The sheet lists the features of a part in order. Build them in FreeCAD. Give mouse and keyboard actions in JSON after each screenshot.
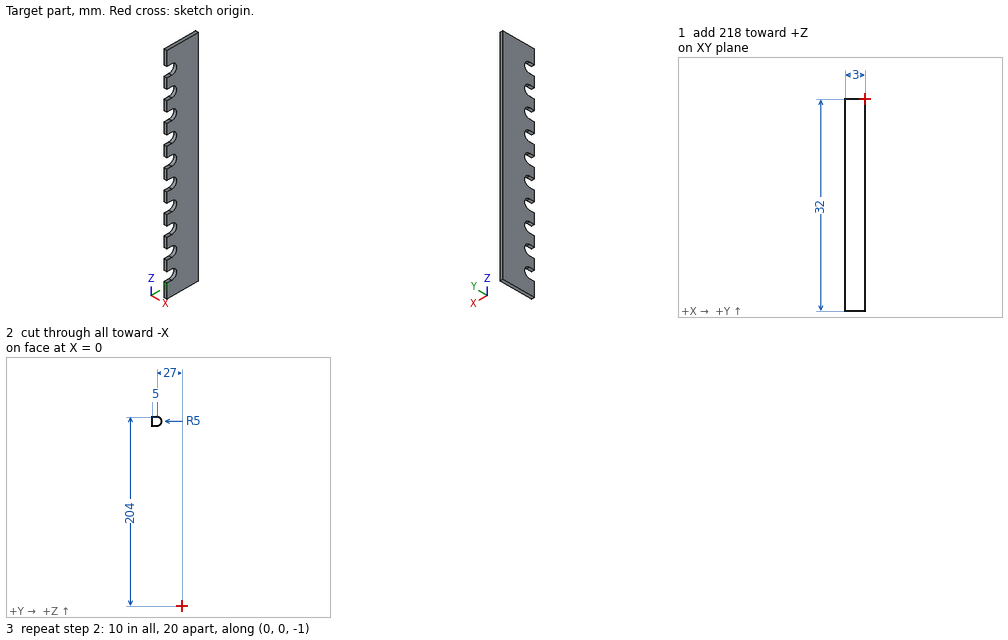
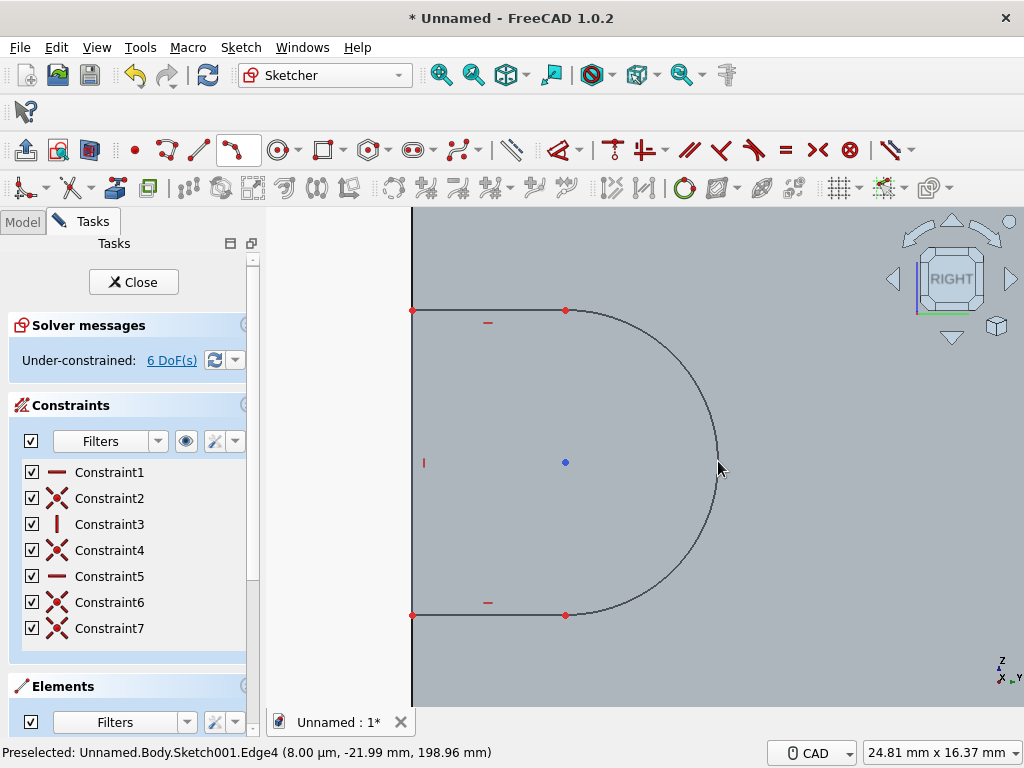
{"action": "left_click", "coordinate": [519, 310]}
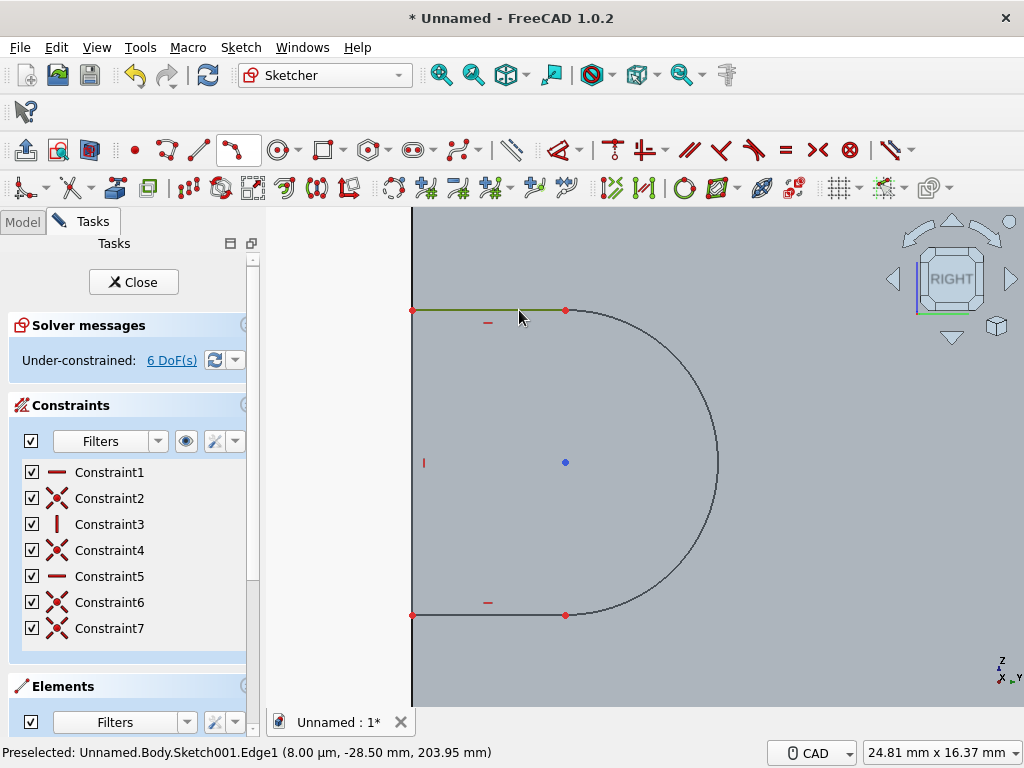
{"action": "left_click", "coordinate": [689, 552]}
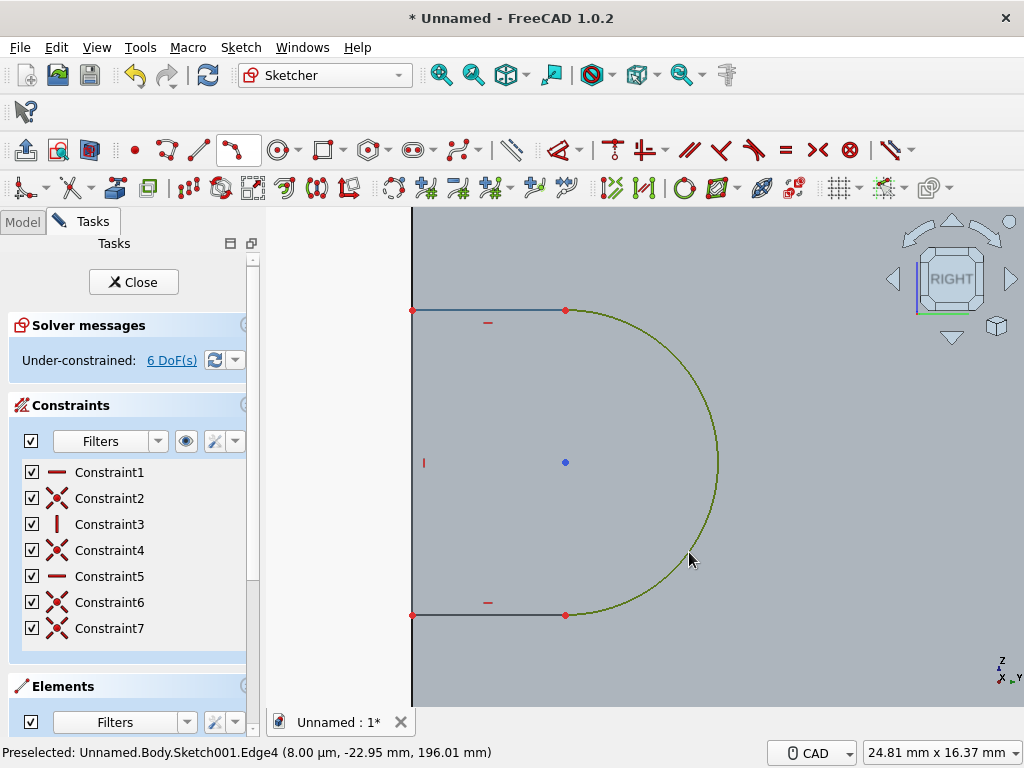
{"action": "left_click", "coordinate": [754, 150]}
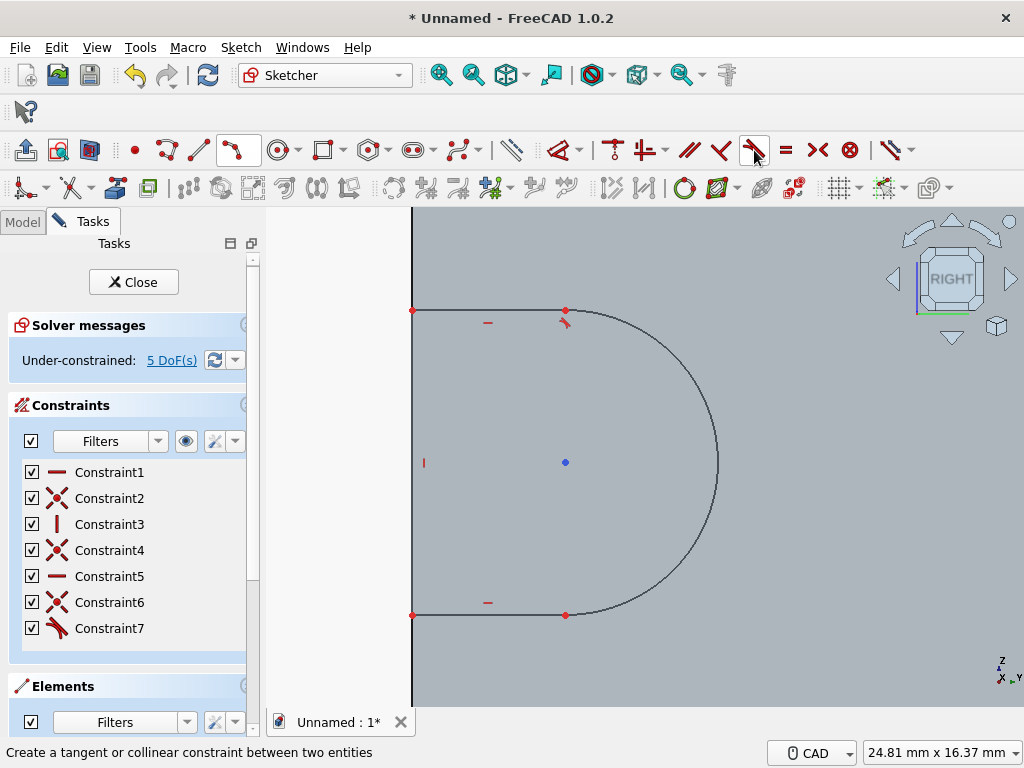
{"action": "left_click", "coordinate": [458, 615]}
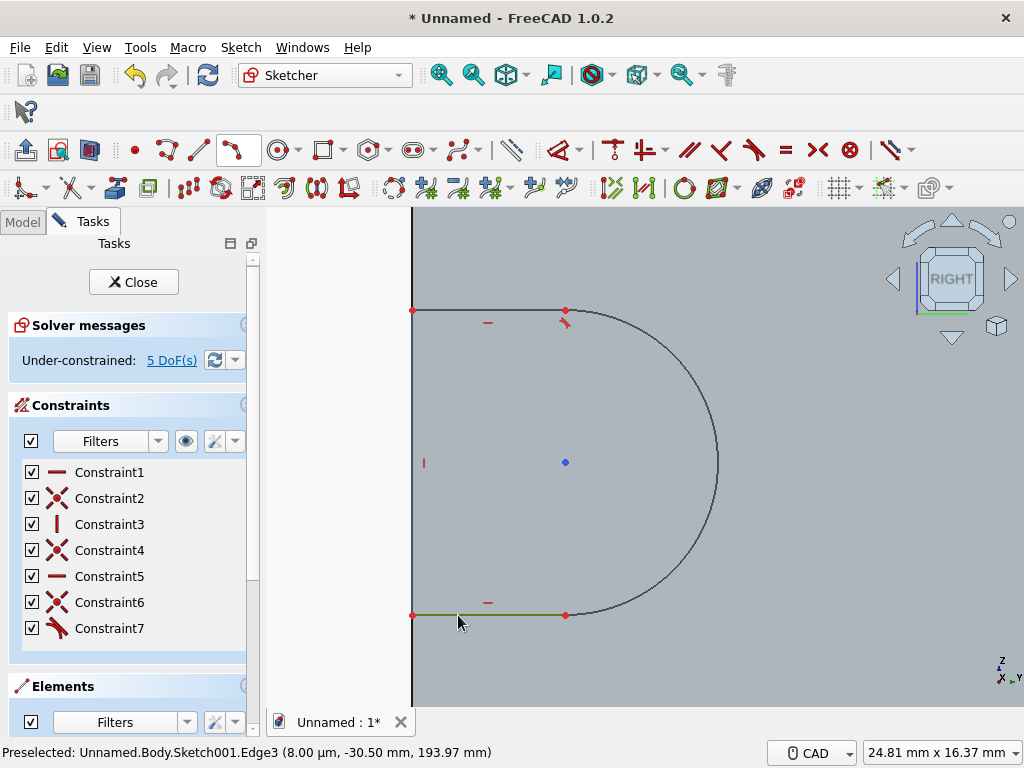
{"action": "left_click", "coordinate": [689, 552]}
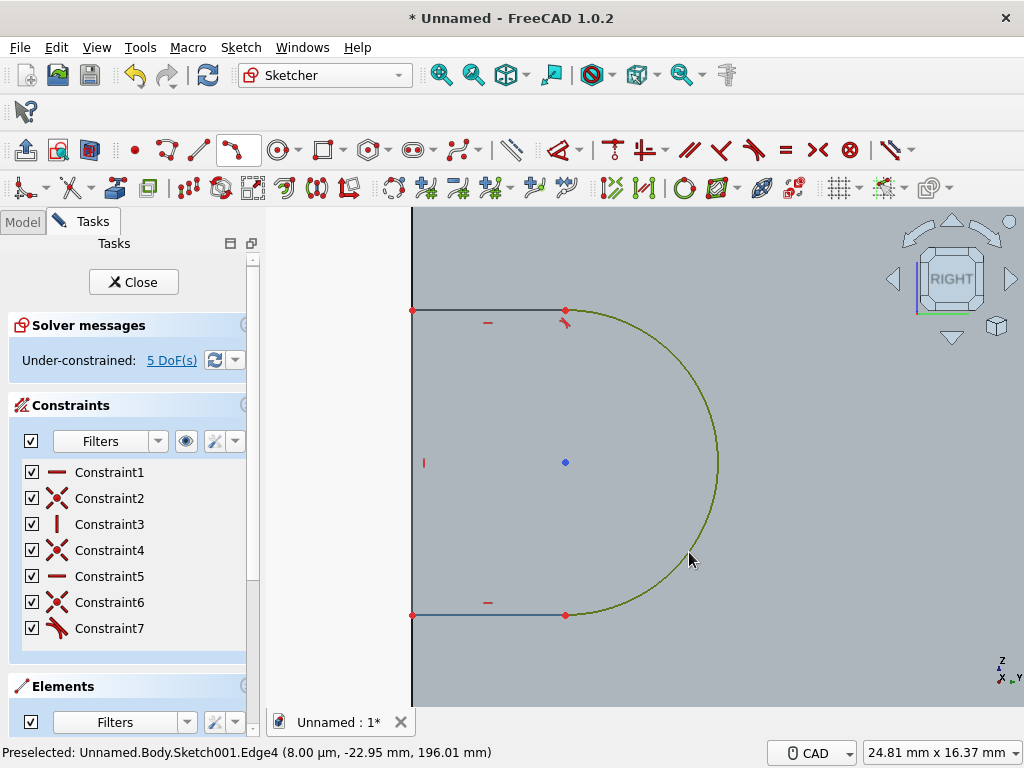
{"action": "left_click", "coordinate": [754, 150]}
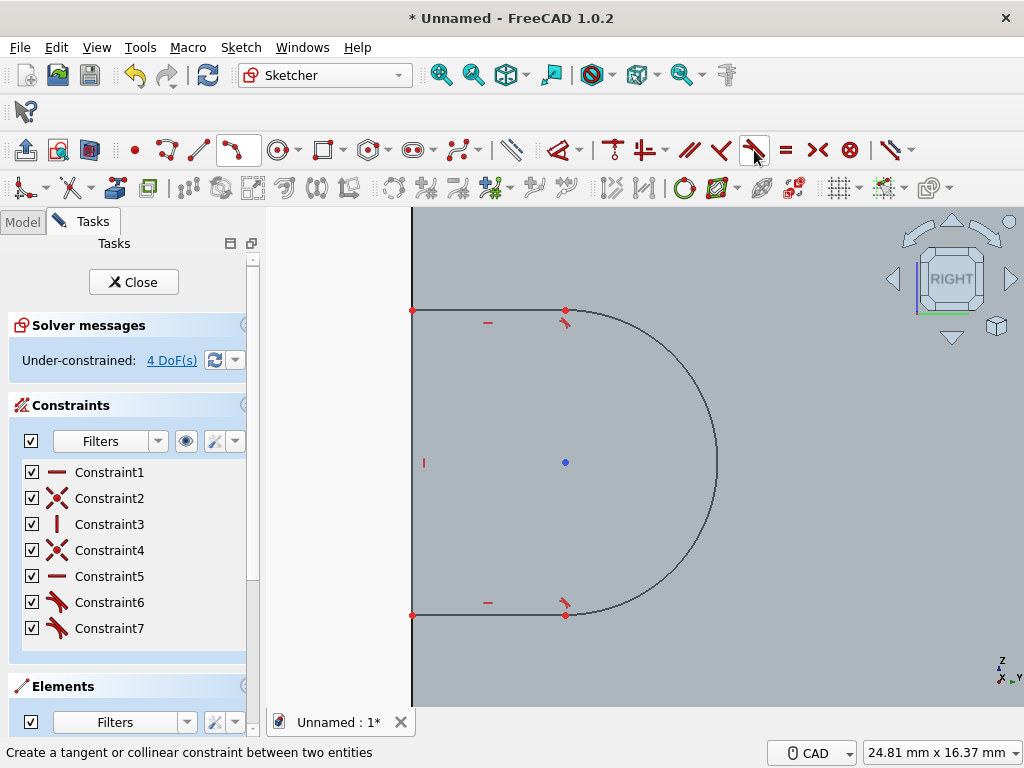
{"action": "left_click", "coordinate": [558, 150]}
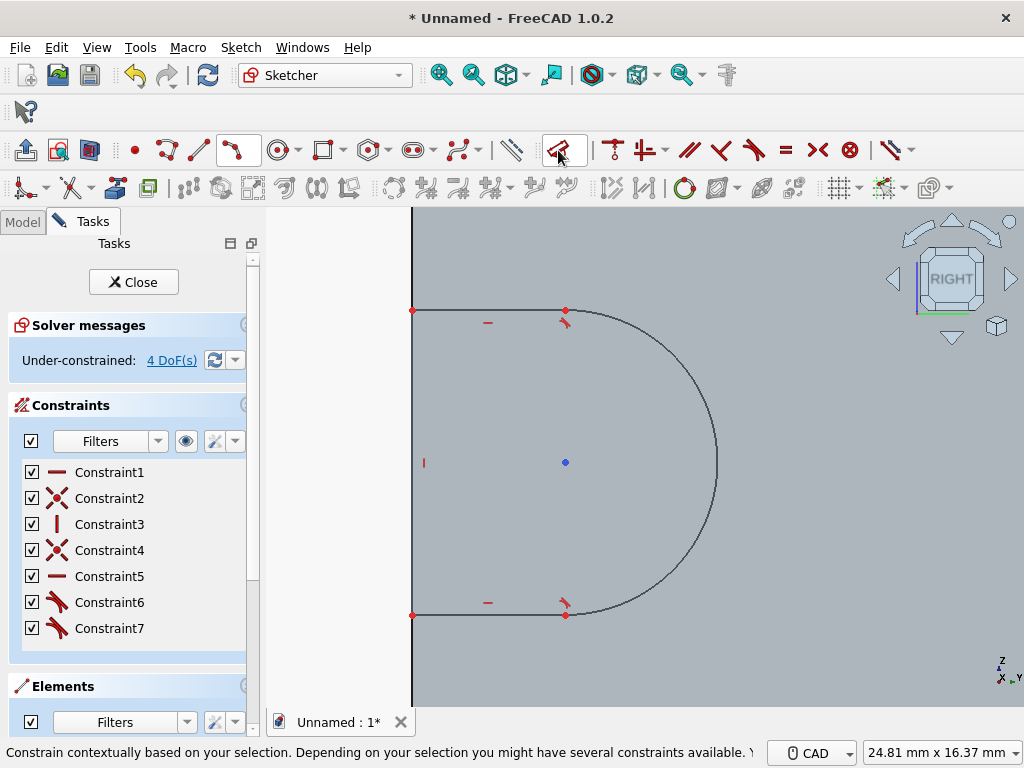
{"action": "left_click", "coordinate": [688, 552]}
{"action": "left_click", "coordinate": [714, 571]}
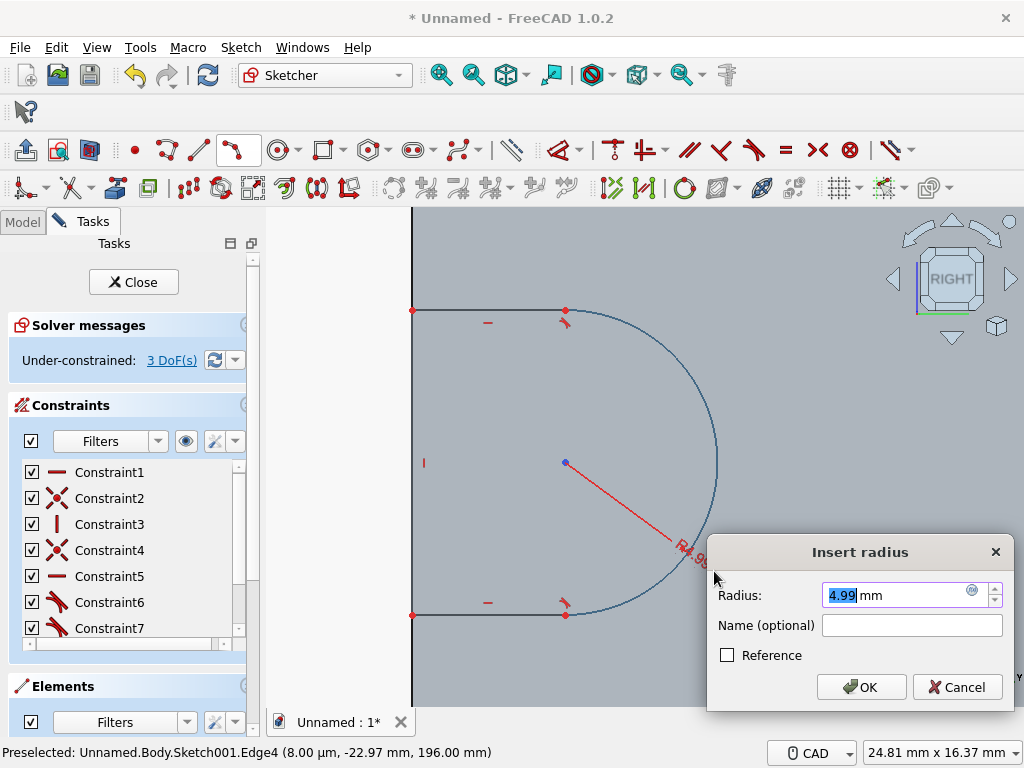
{"action": "type", "text": "5"}
{"action": "key", "text": "Return"}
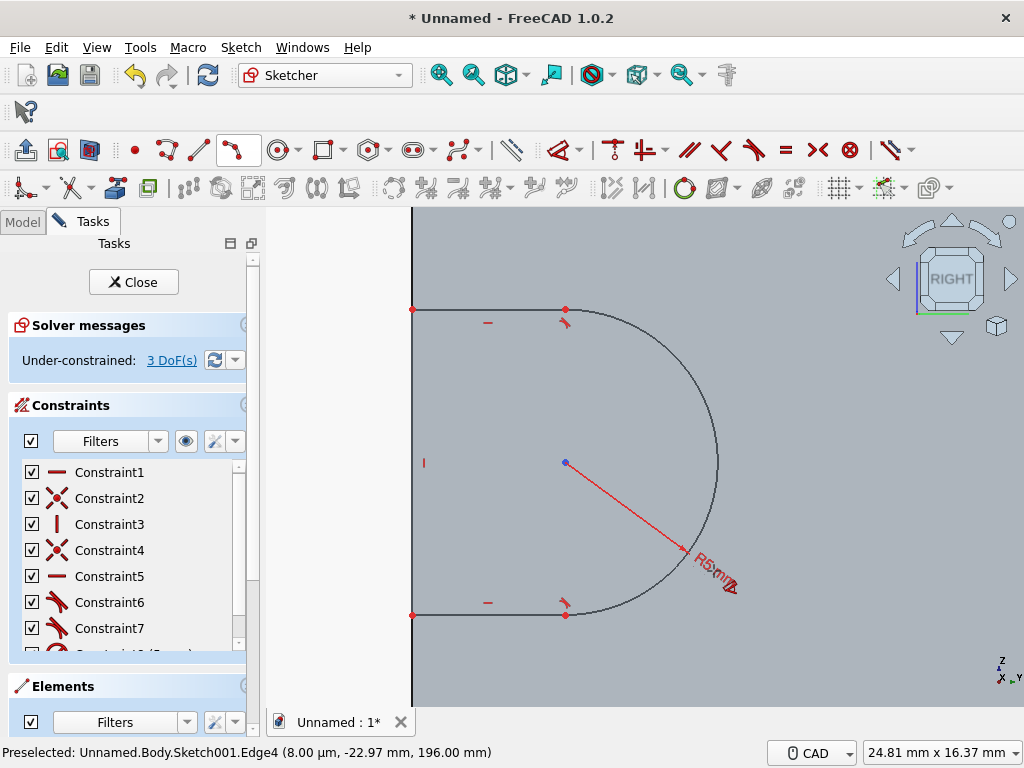
{"action": "left_click", "coordinate": [519, 310]}
{"action": "left_click", "coordinate": [489, 276]}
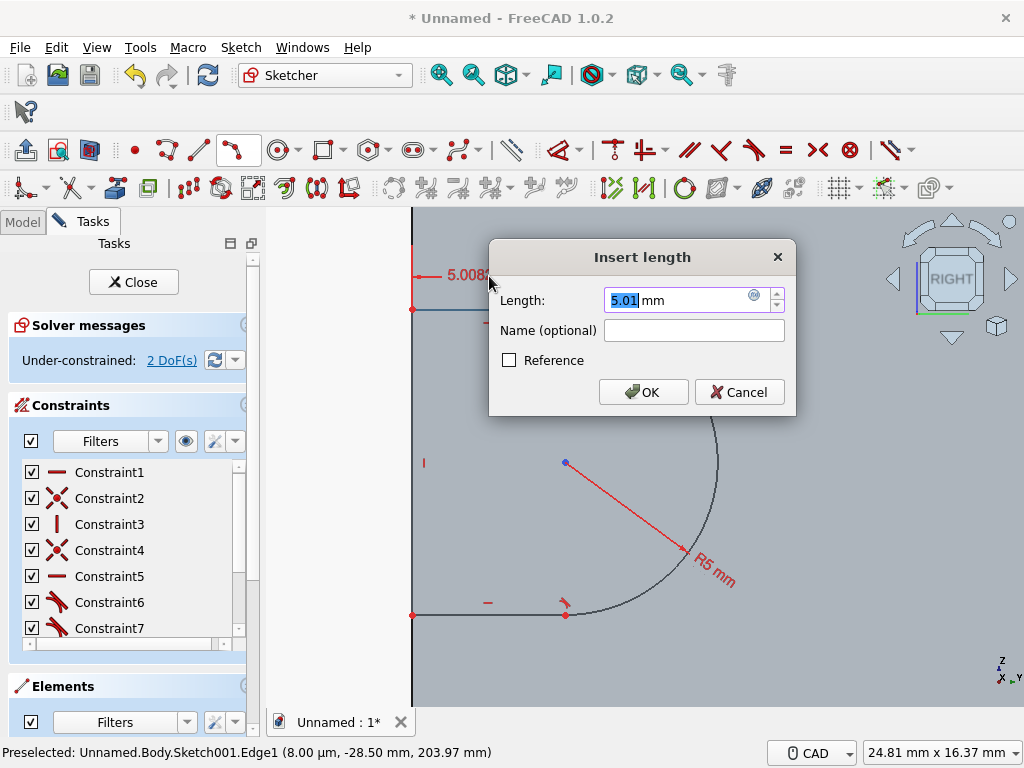
{"action": "type", "text": "5"}
{"action": "key", "text": "Return"}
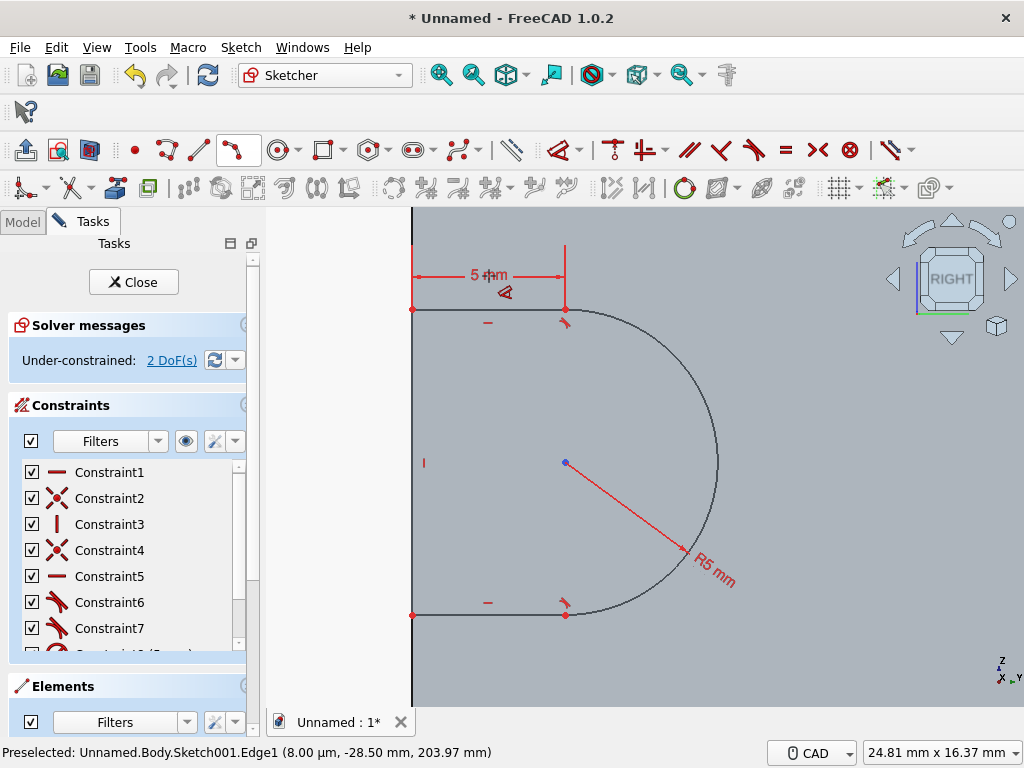
{"action": "left_click", "coordinate": [565, 310]}
{"action": "left_click", "coordinate": [712, 276]}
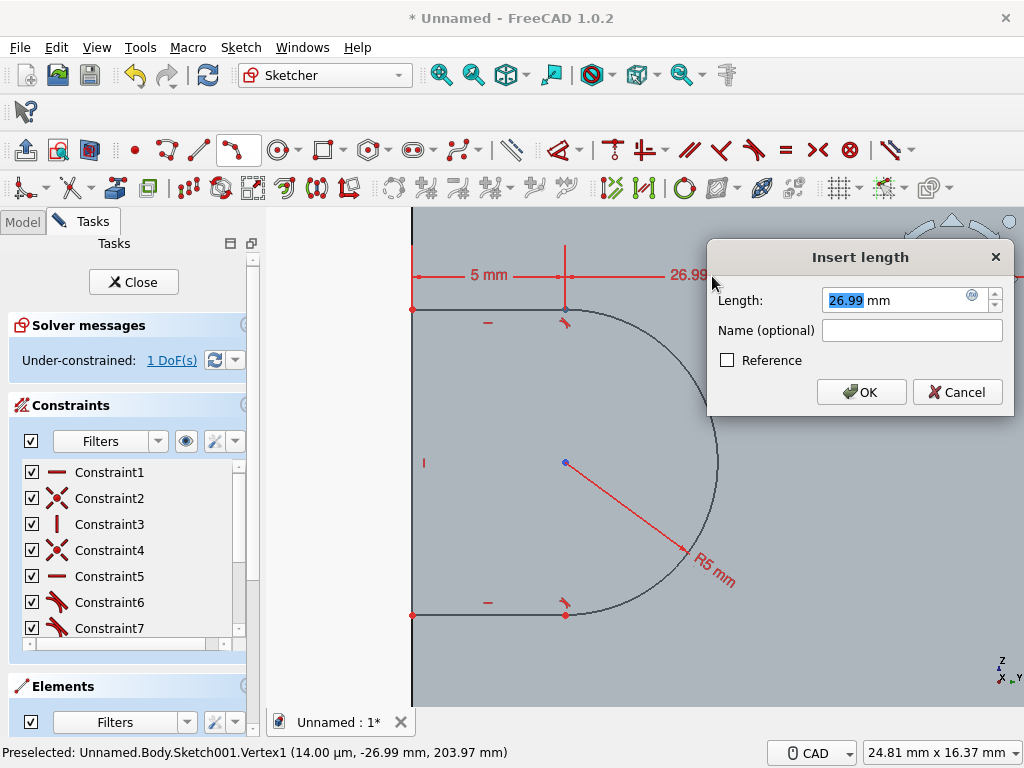
{"action": "type", "text": "27"}
{"action": "key", "text": "Return"}